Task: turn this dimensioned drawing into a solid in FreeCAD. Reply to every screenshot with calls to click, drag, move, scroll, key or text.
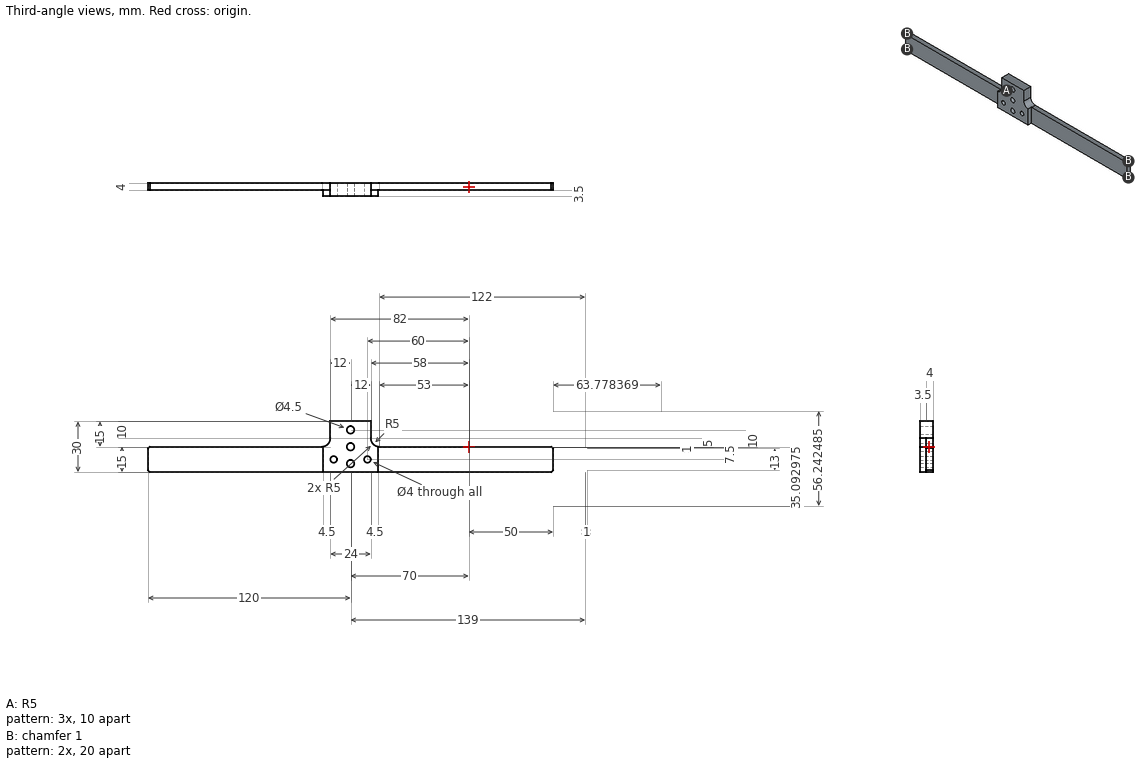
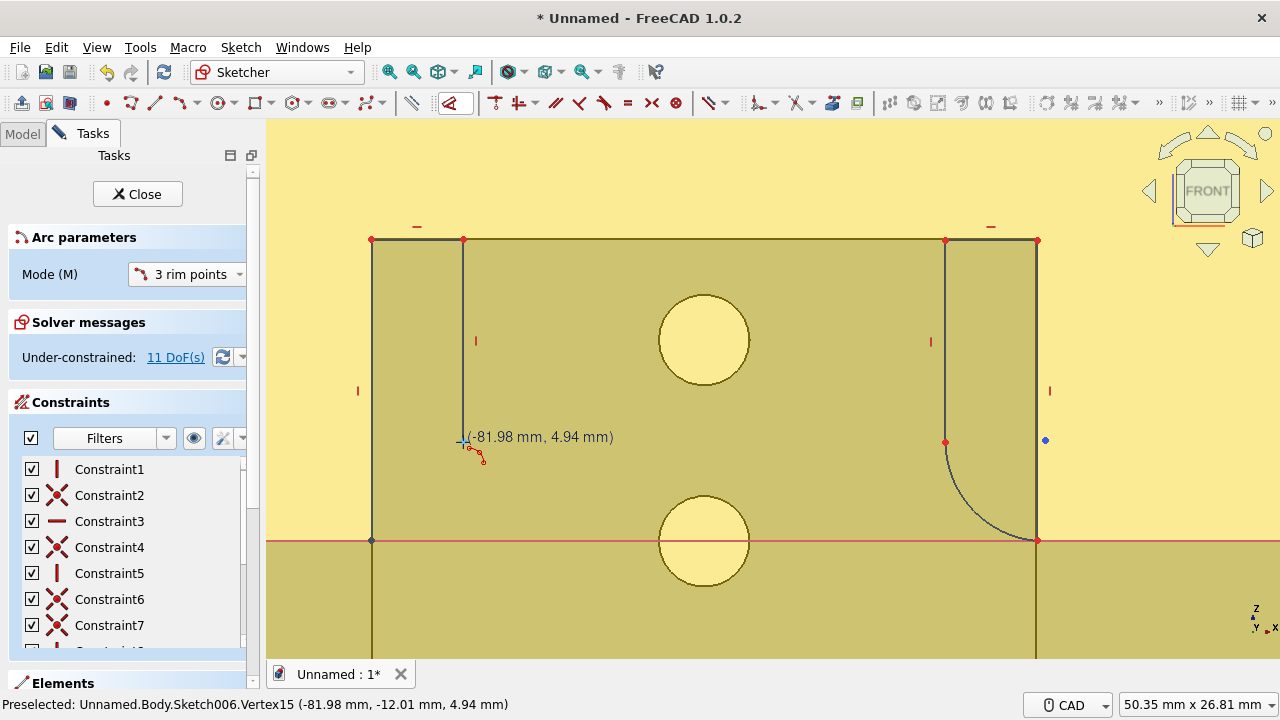
scroll(372, 541, up, 18)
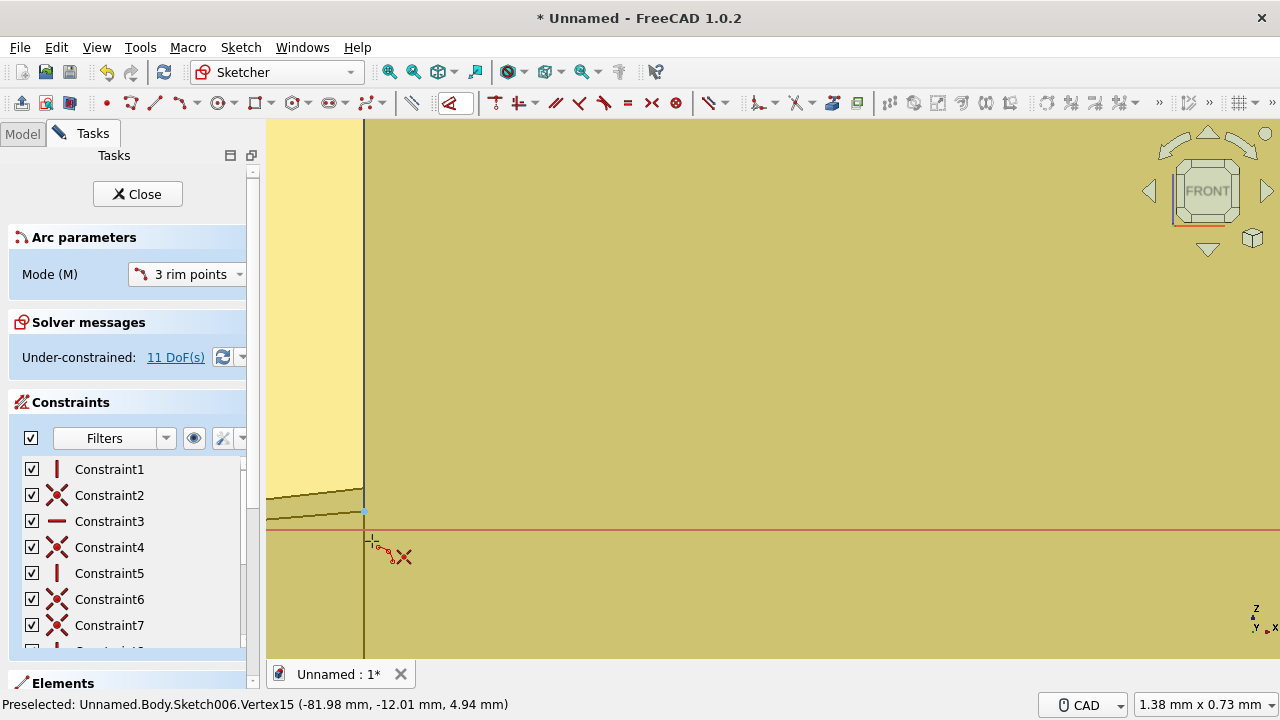
click(364, 512)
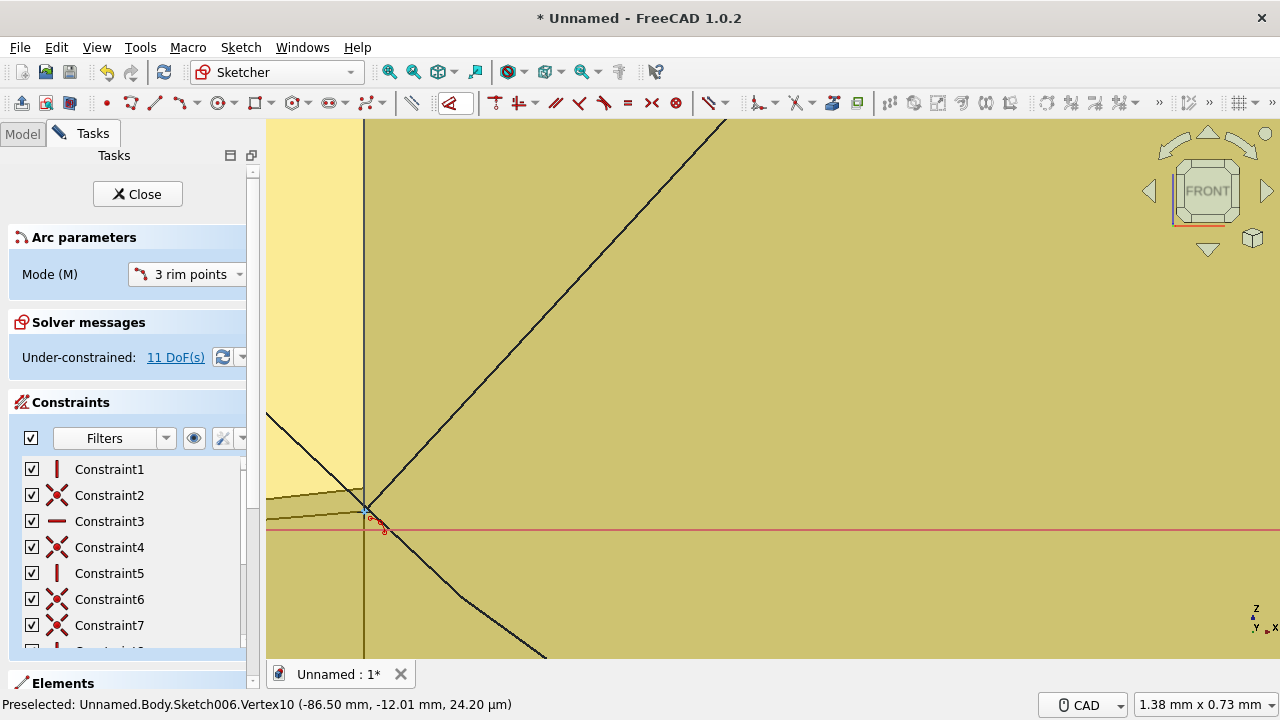
scroll(372, 541, down, 18)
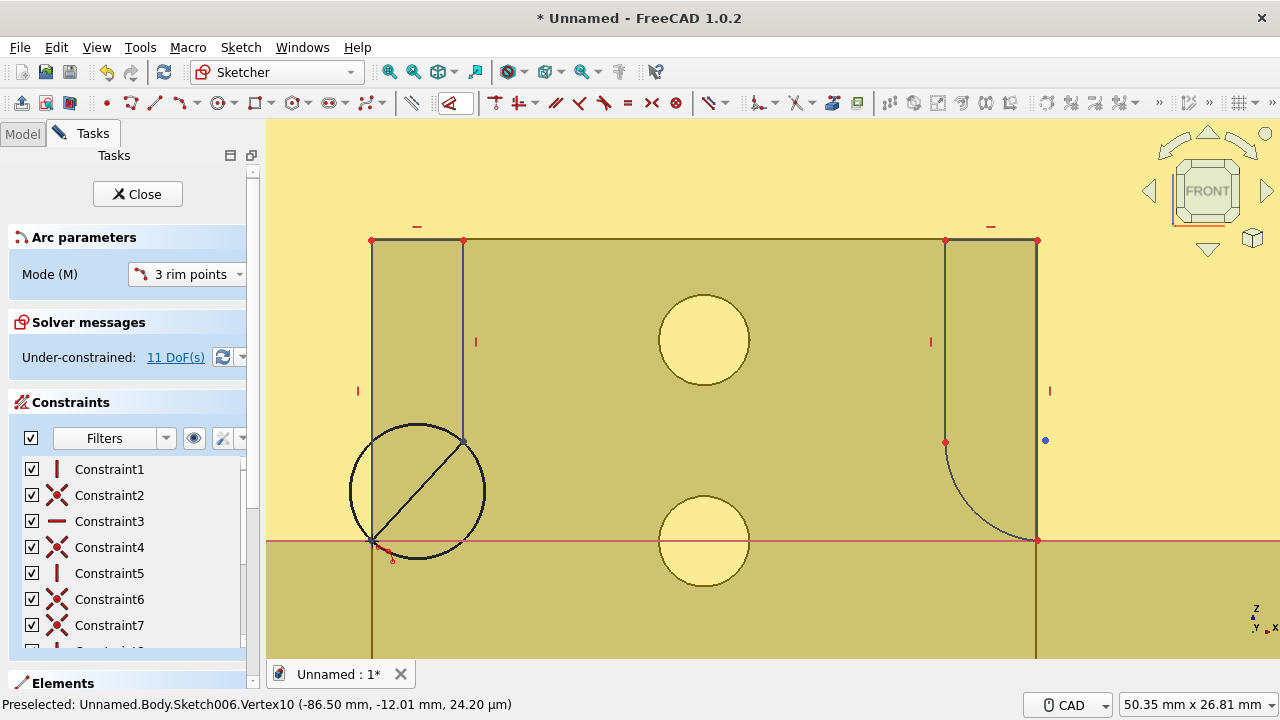
click(436, 508)
key(Escape)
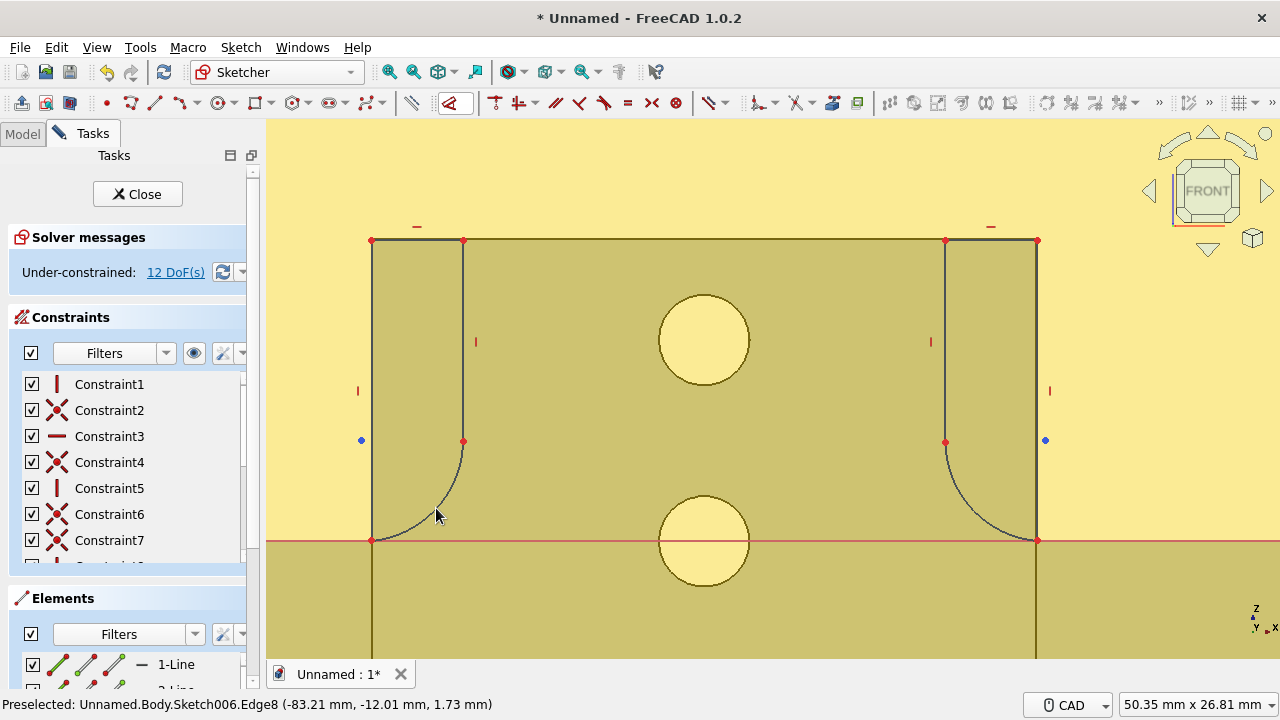
click(945, 382)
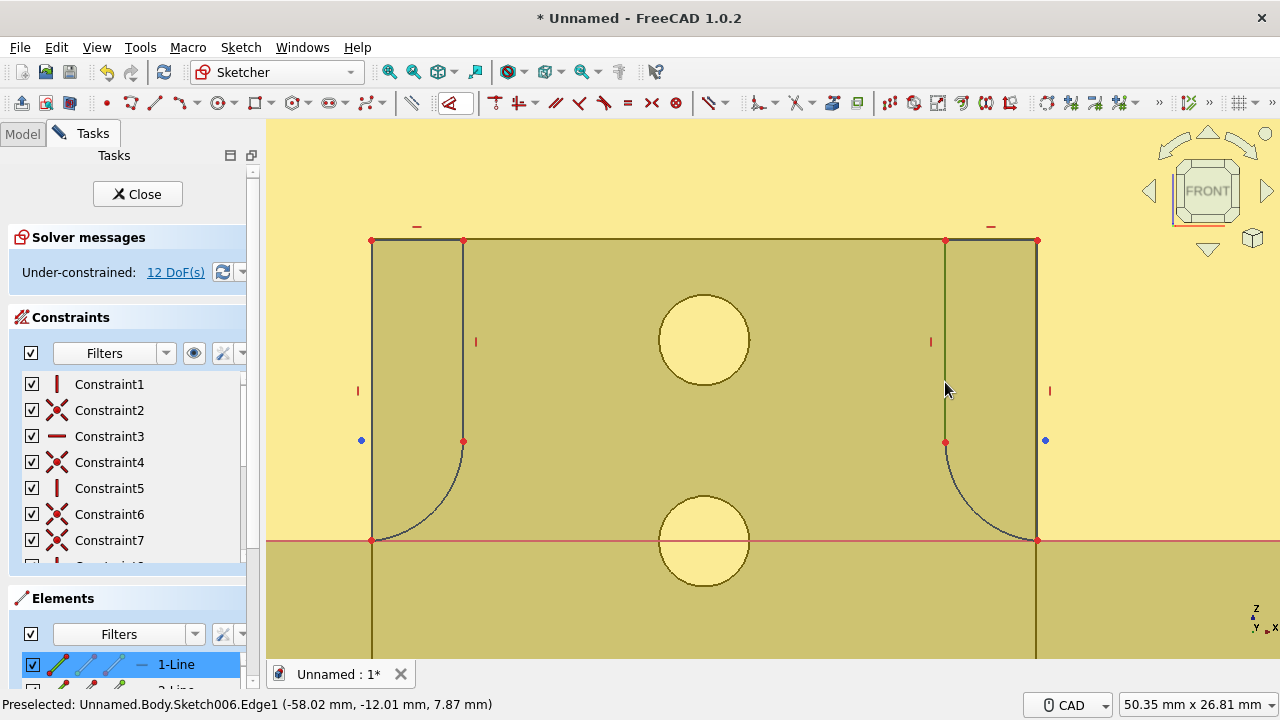
click(956, 485)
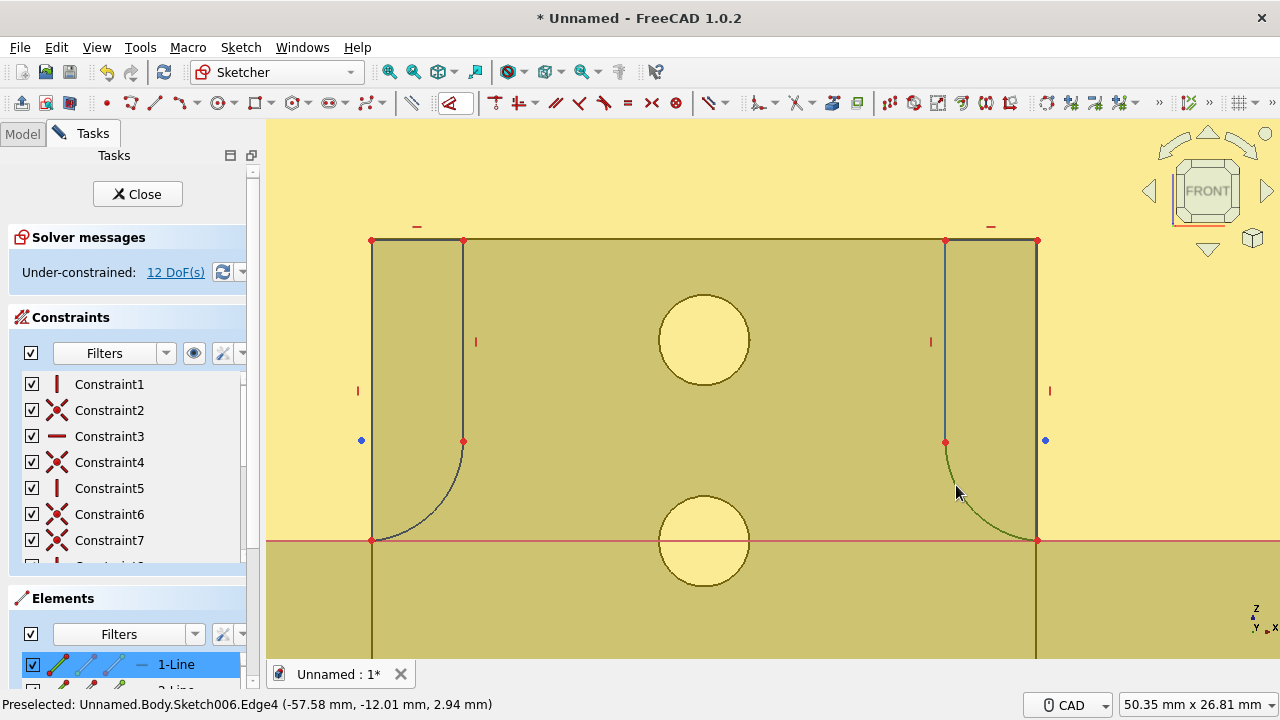
click(604, 104)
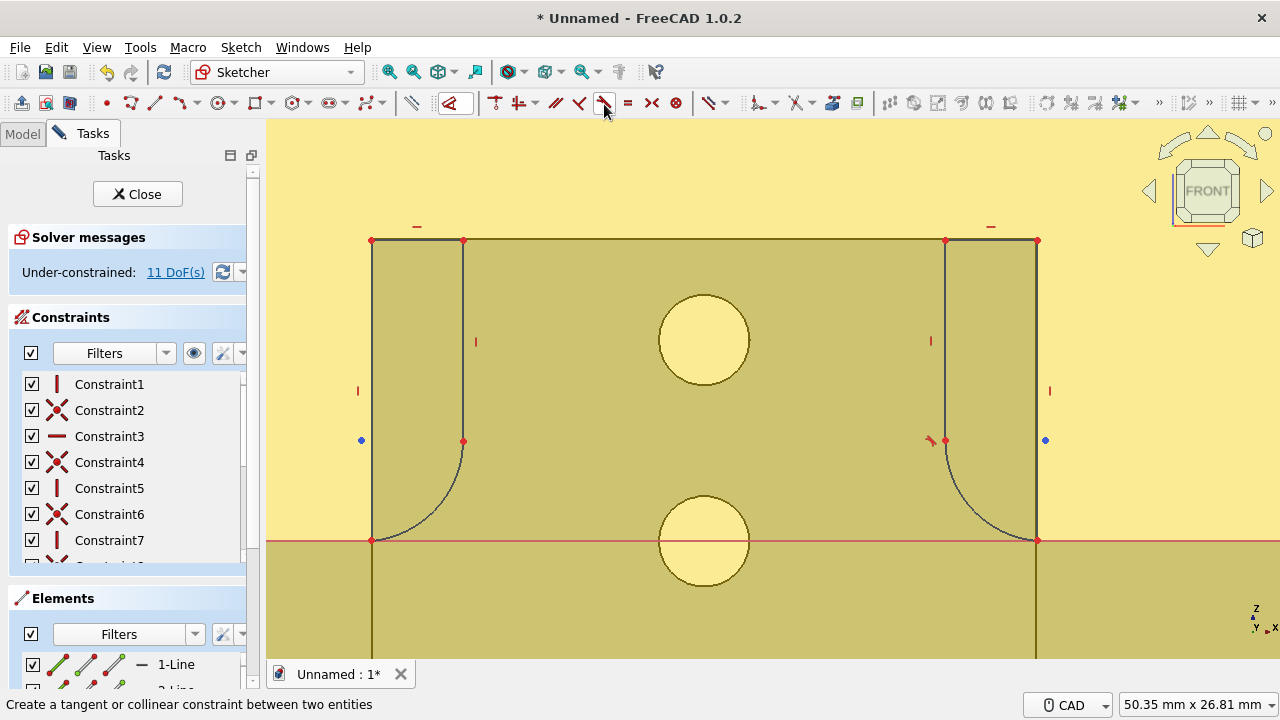
click(463, 301)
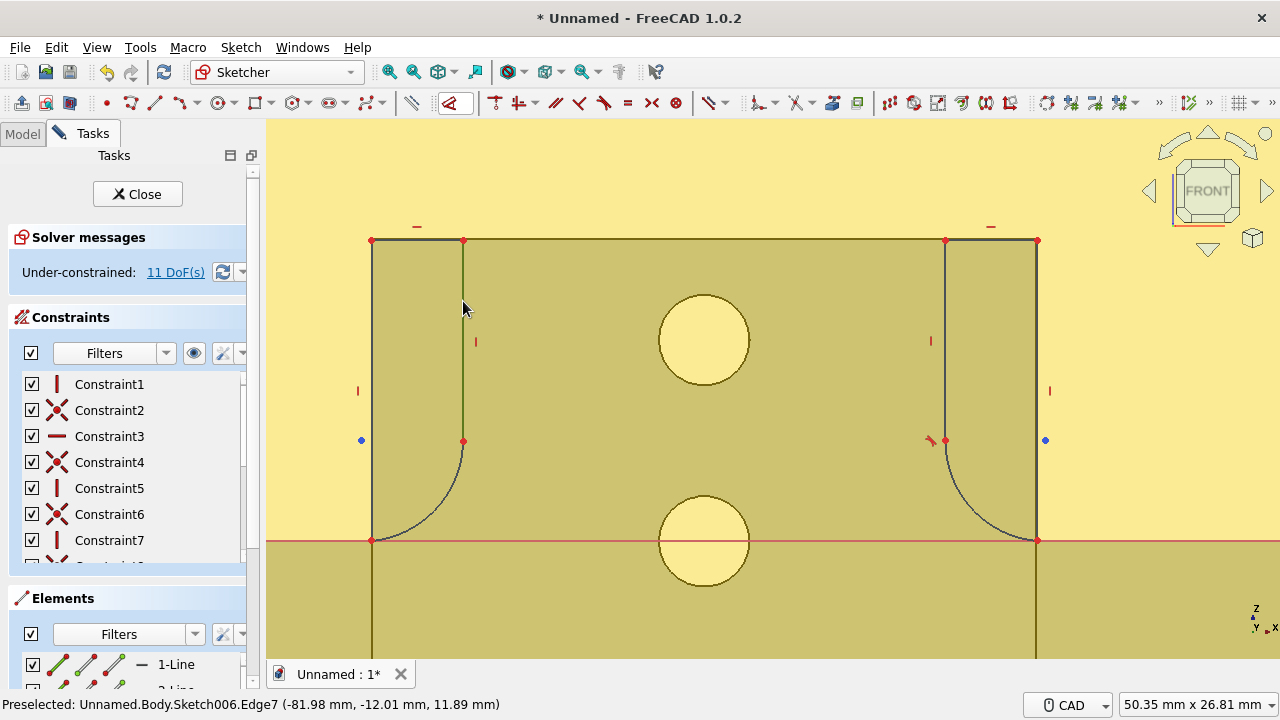
click(413, 527)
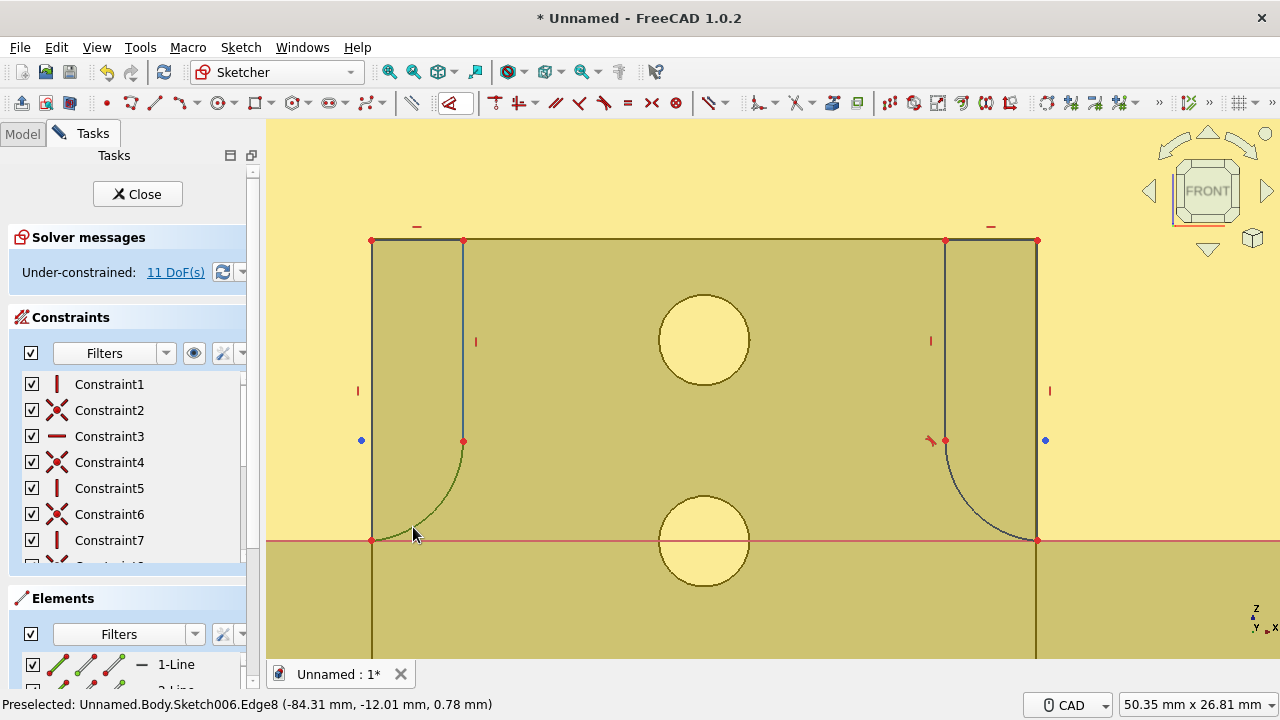
click(604, 104)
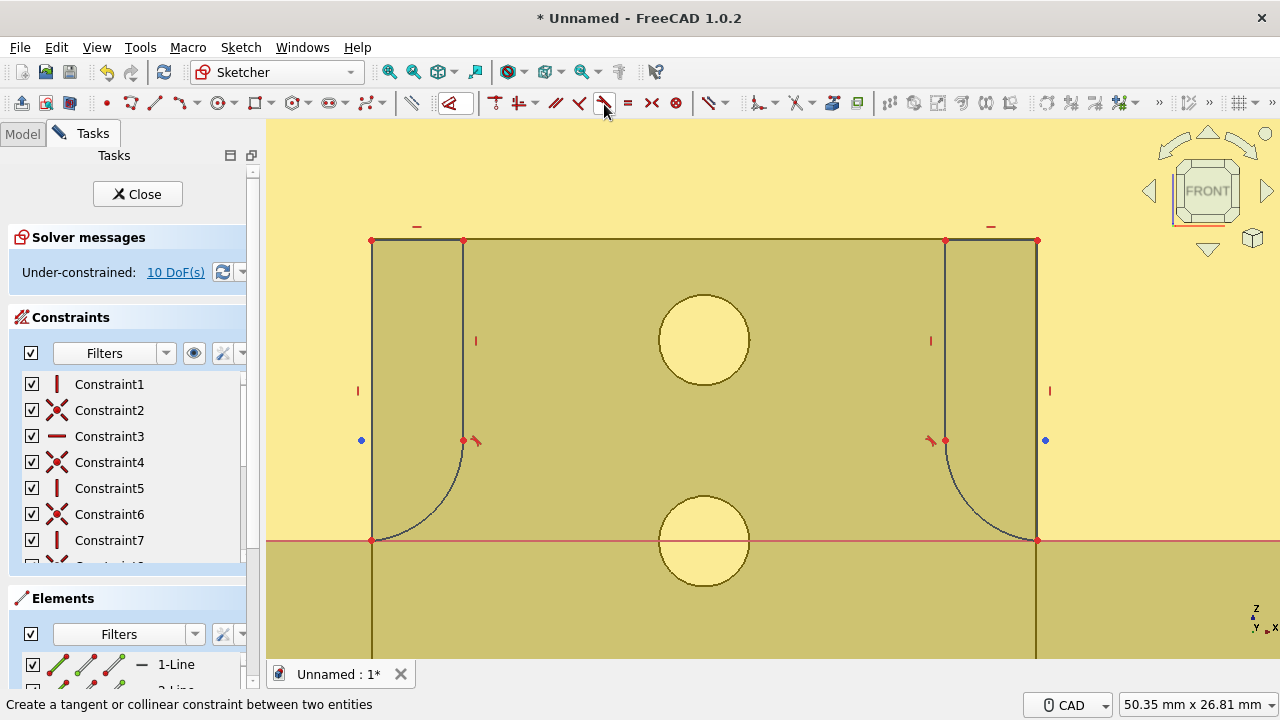
click(955, 484)